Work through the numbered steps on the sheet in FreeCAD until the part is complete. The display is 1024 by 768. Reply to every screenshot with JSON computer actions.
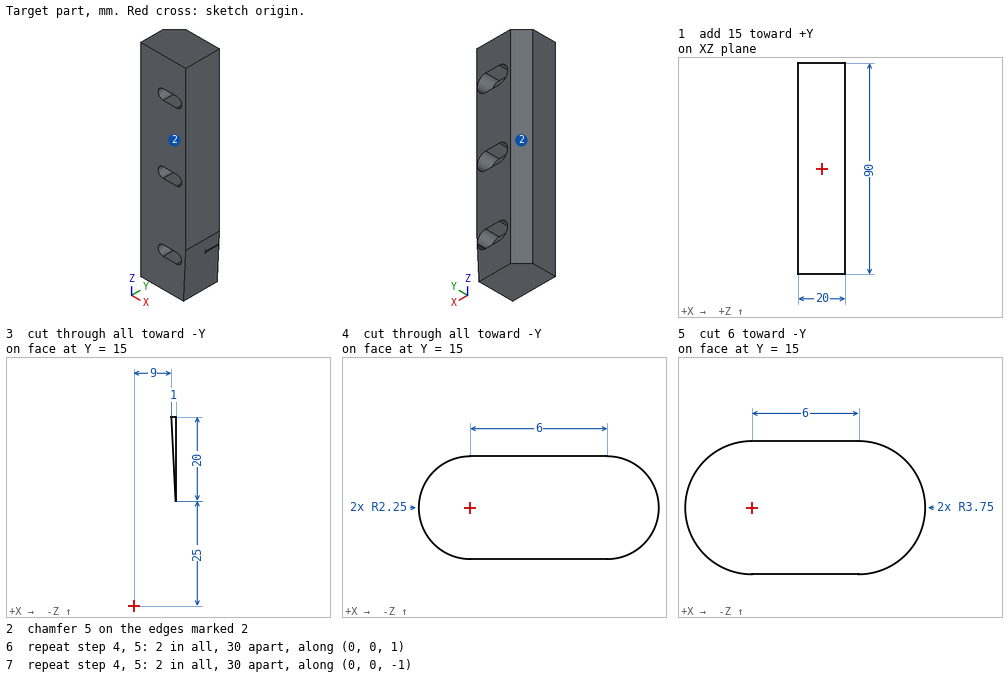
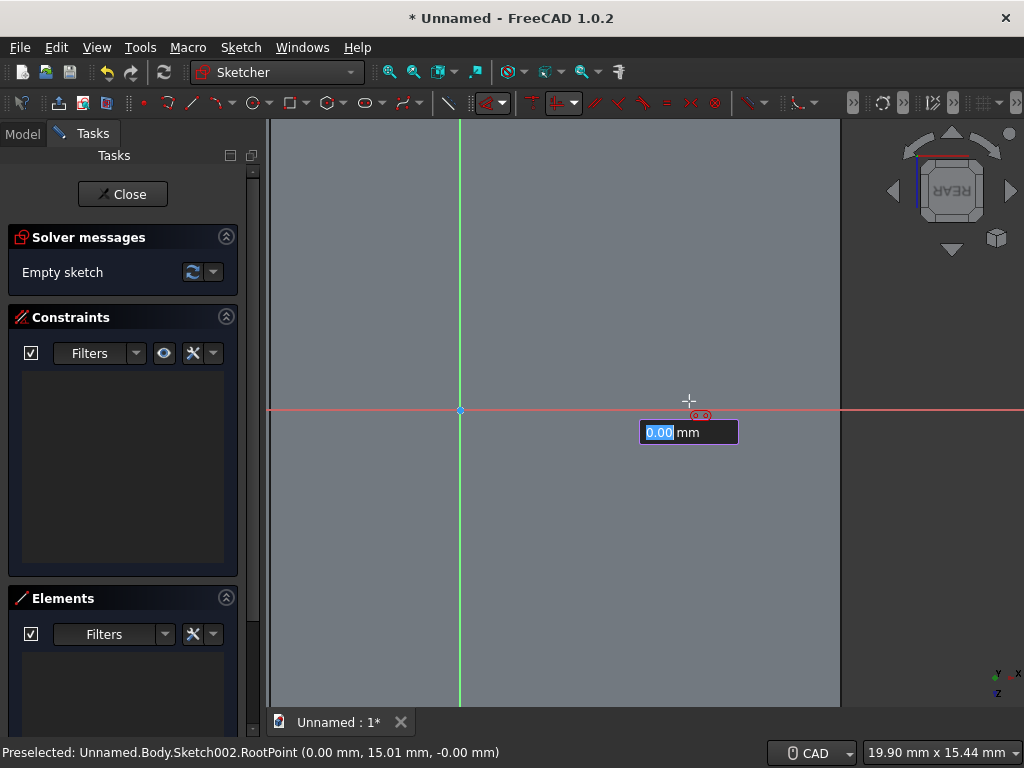
{"action": "left_click", "coordinate": [575, 325]}
{"action": "key", "text": "Escape"}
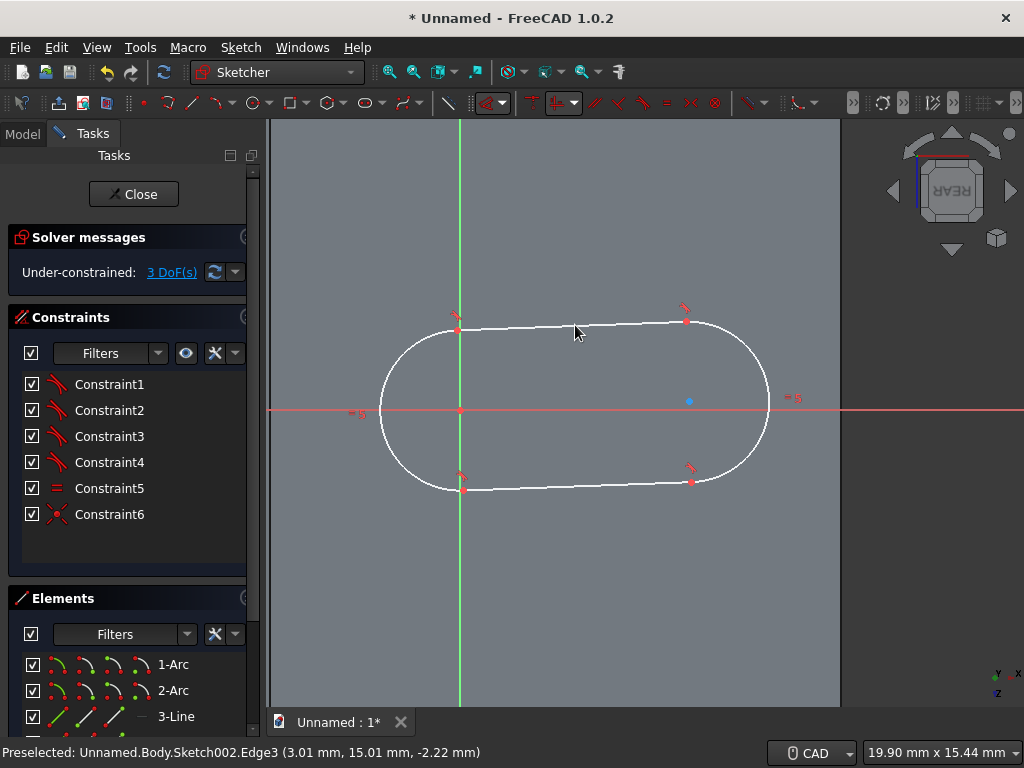
{"action": "left_click", "coordinate": [526, 328]}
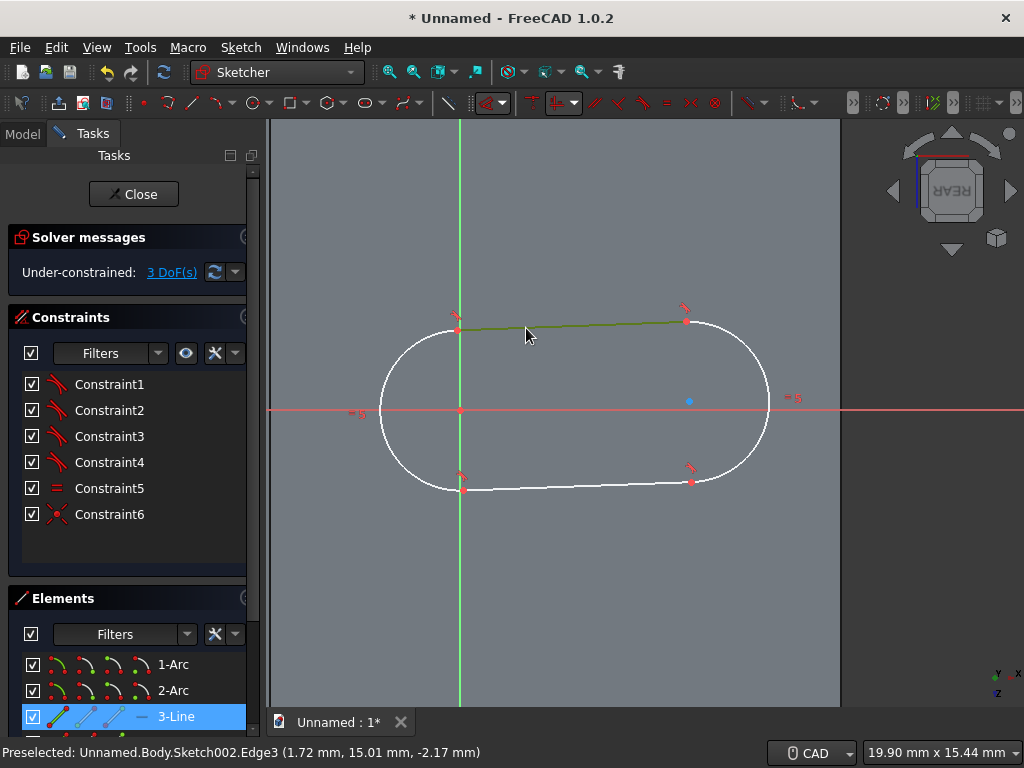
{"action": "key", "text": "h"}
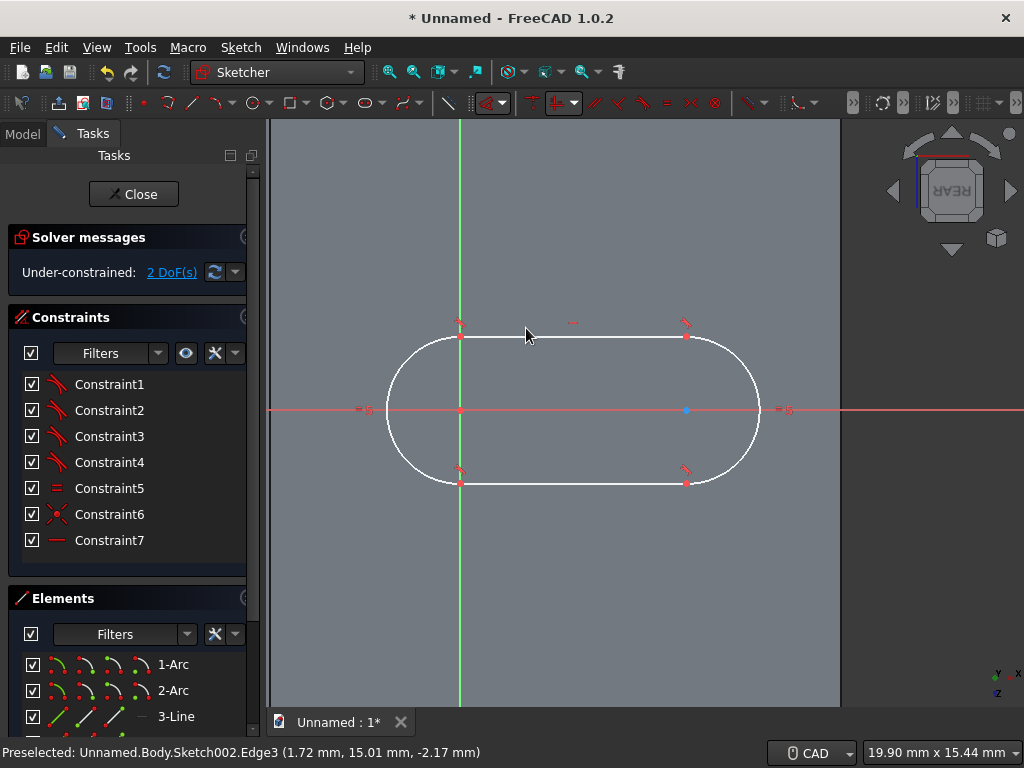
{"action": "left_click", "coordinate": [401, 367]}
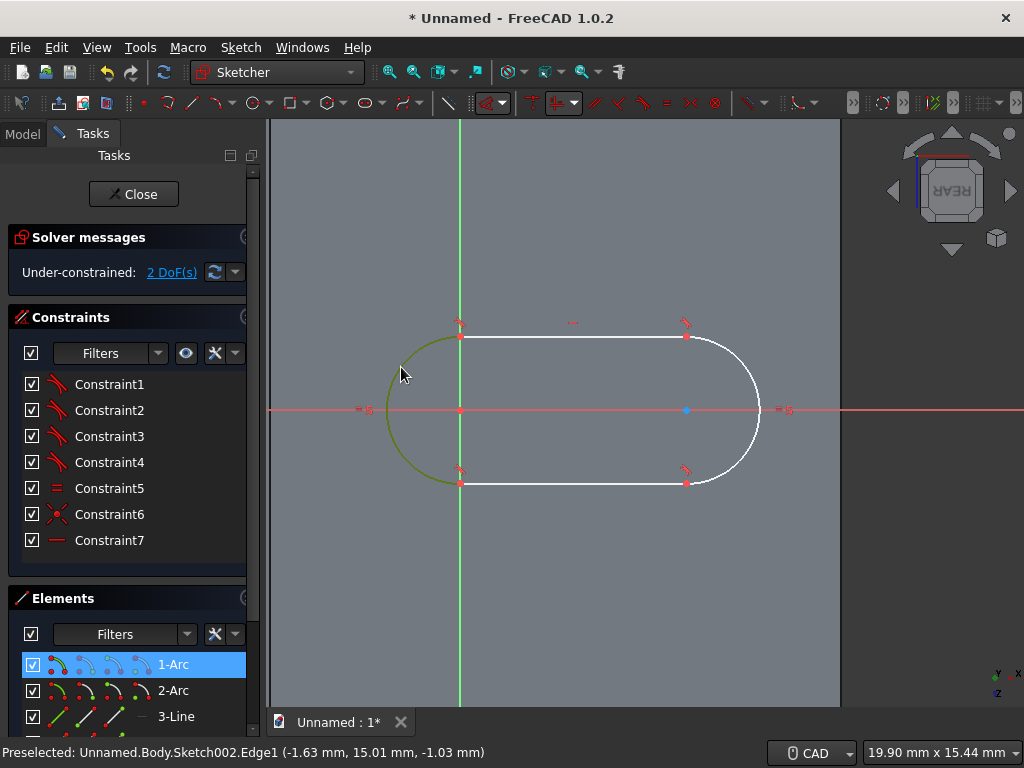
{"action": "key", "text": "k r"}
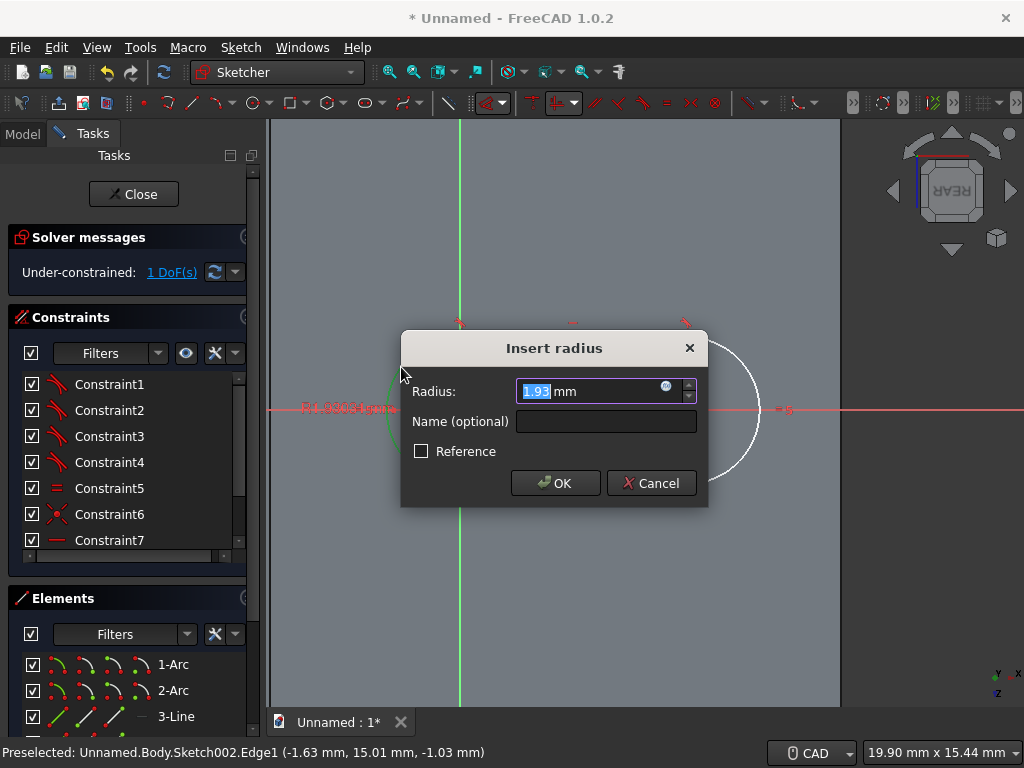
{"action": "type", "text": "2.25"}
{"action": "key", "text": "Return"}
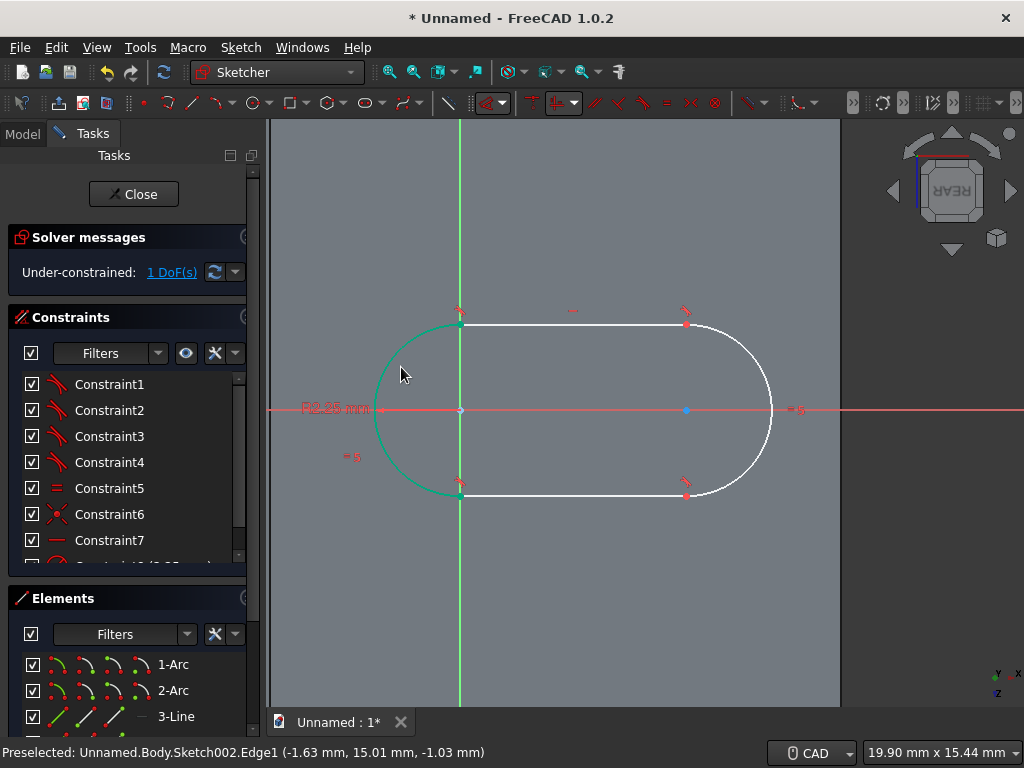
{"action": "left_click", "coordinate": [528, 325]}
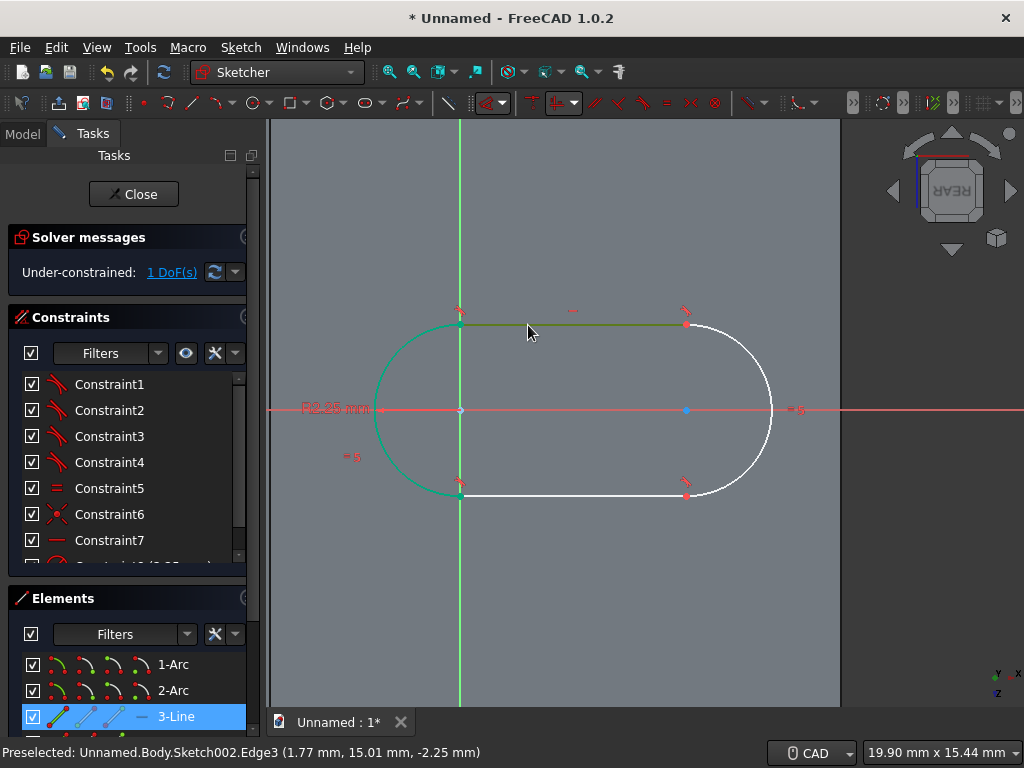
{"action": "left_click", "coordinate": [504, 104]}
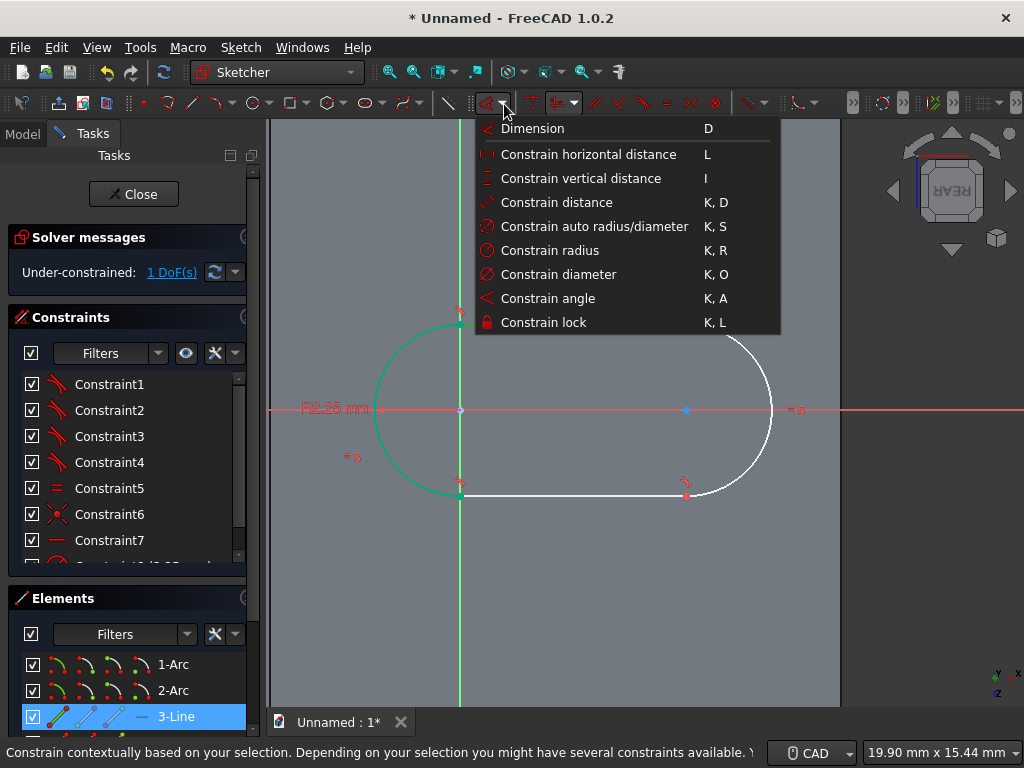
{"action": "left_click", "coordinate": [628, 154]}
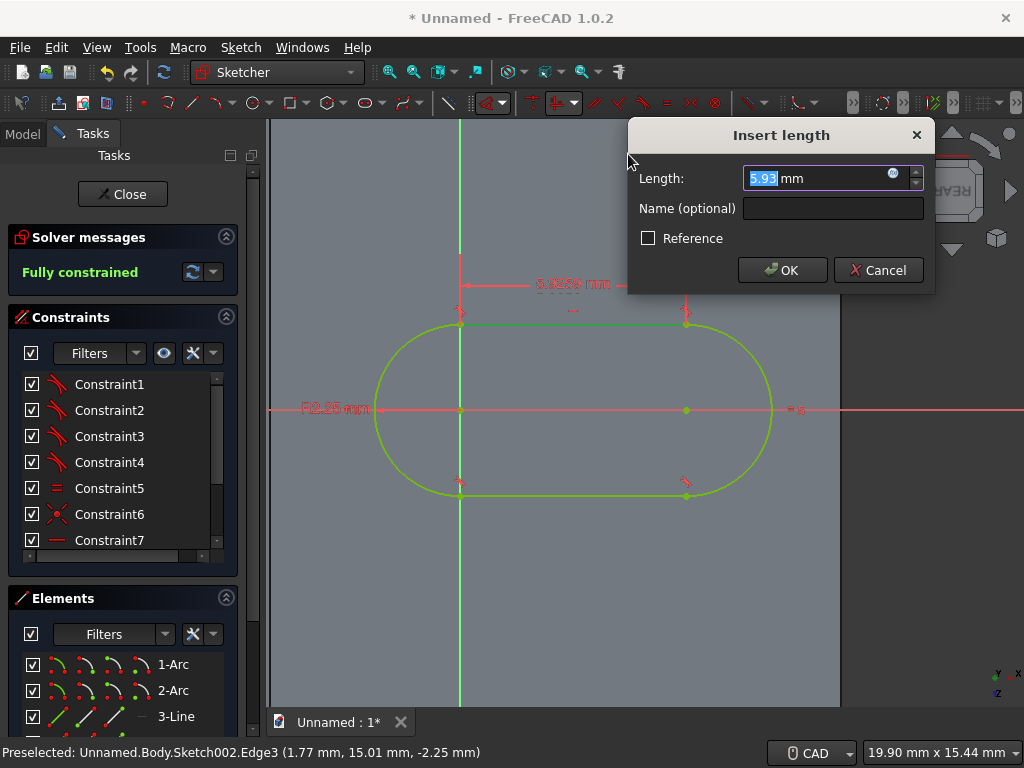
{"action": "type", "text": "6"}
{"action": "key", "text": "Return"}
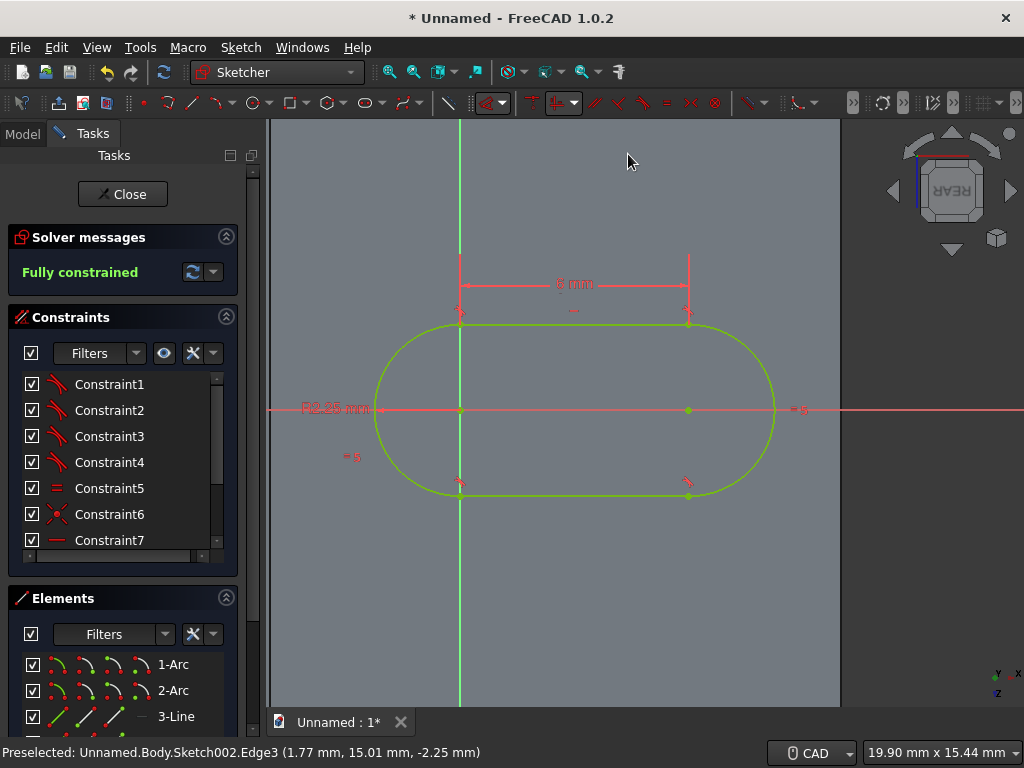
{"action": "left_click", "coordinate": [123, 194]}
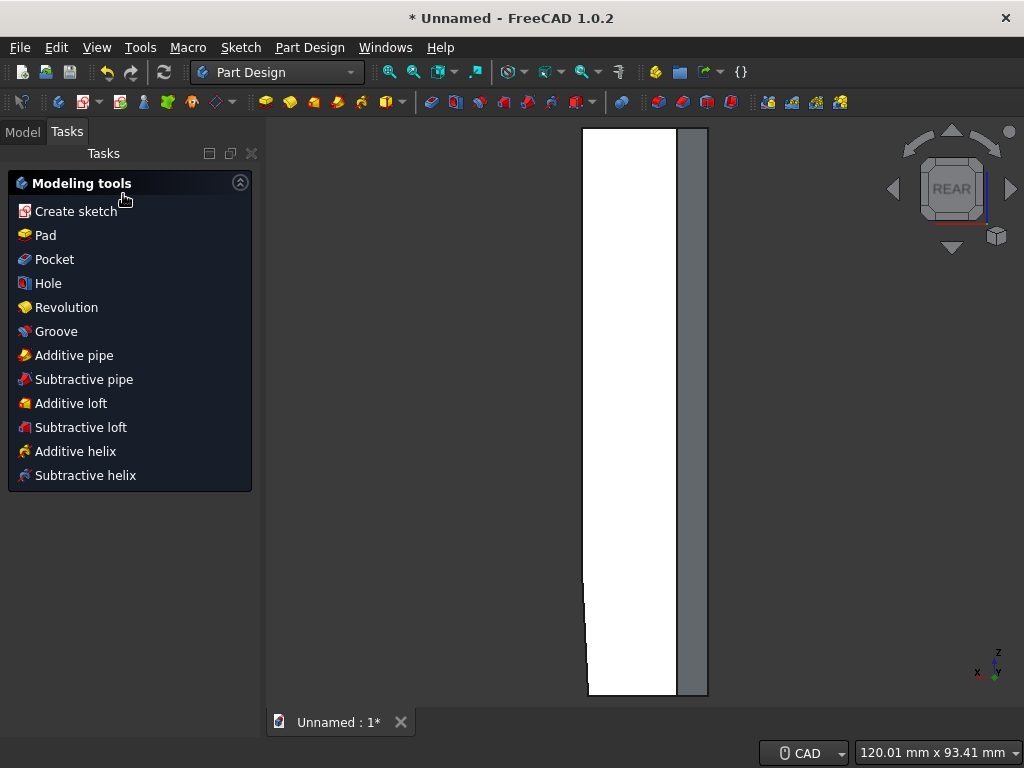
{"action": "left_click", "coordinate": [432, 102]}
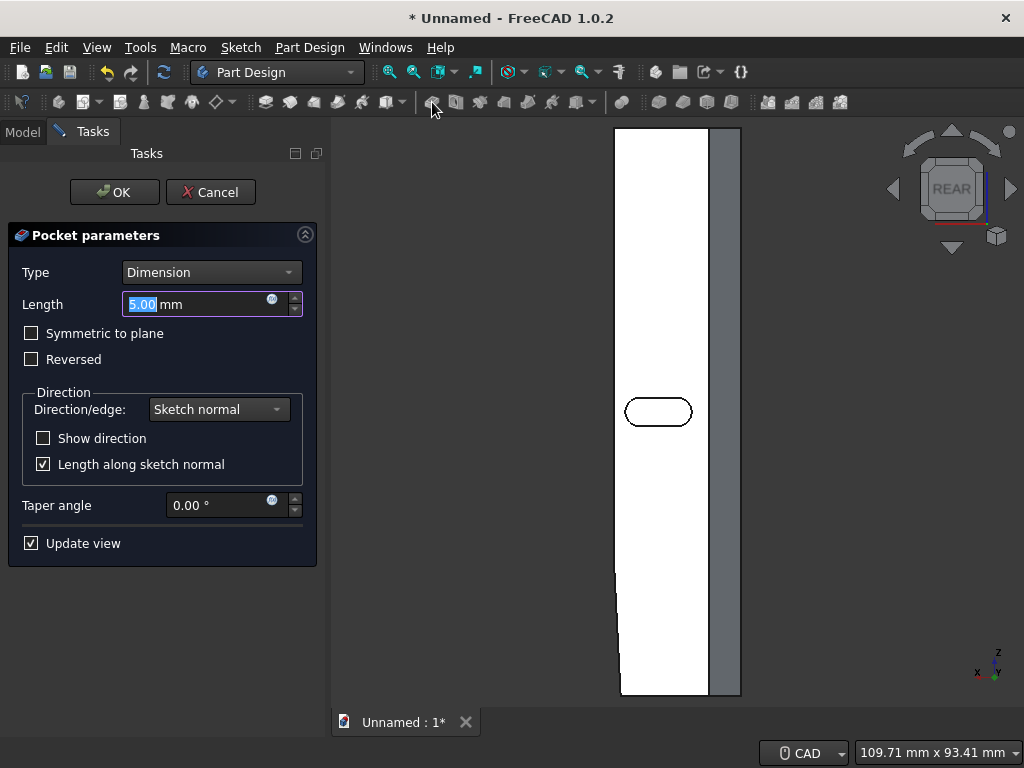
{"action": "left_click", "coordinate": [212, 272]}